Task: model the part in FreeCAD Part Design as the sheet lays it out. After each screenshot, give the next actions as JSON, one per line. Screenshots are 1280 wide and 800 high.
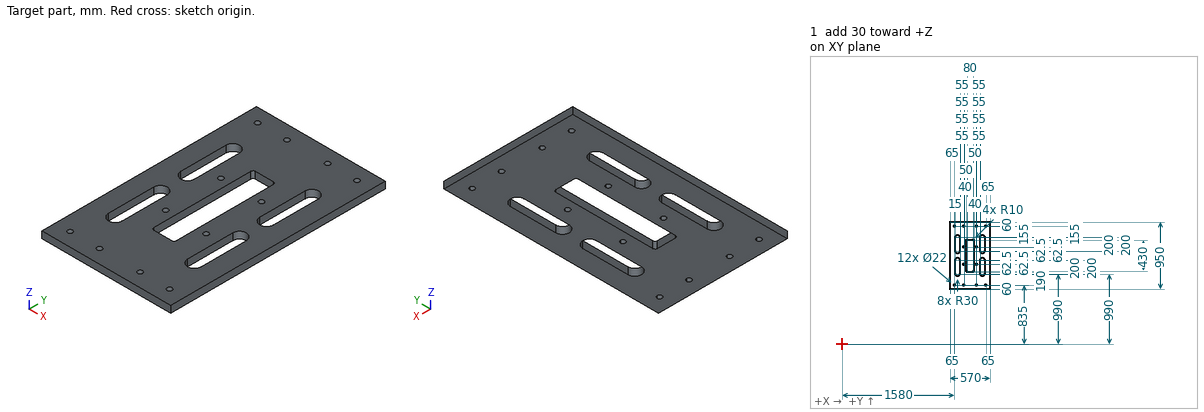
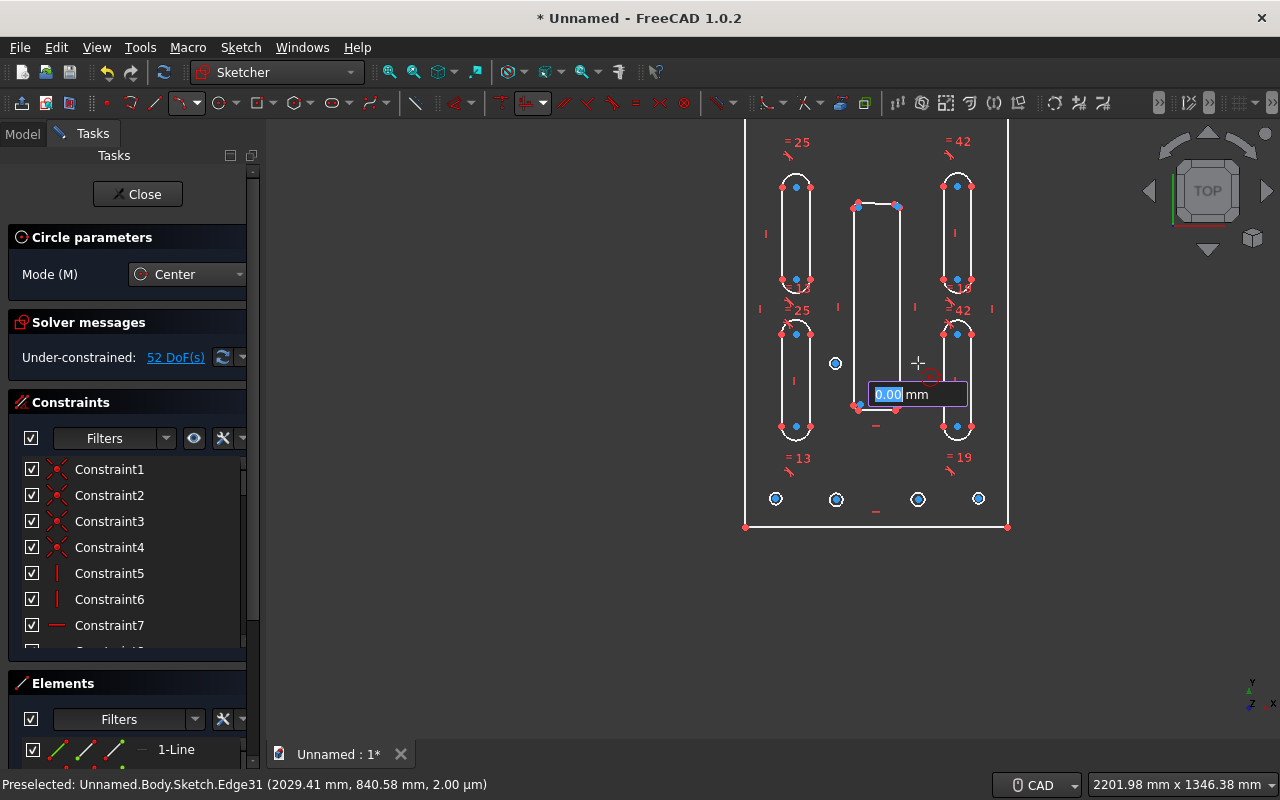
{"action": "scroll", "coordinate": [922, 359], "scroll_direction": "up", "scroll_amount": 6}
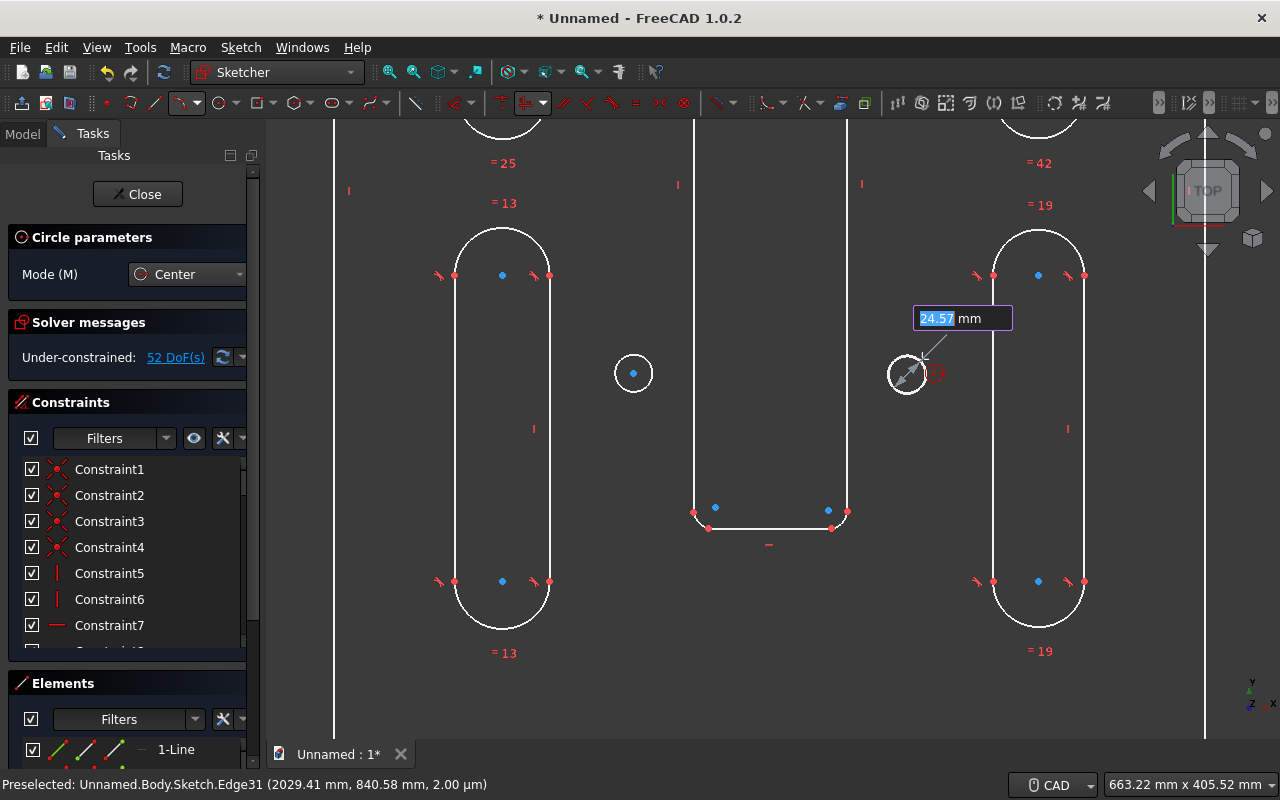
{"action": "left_click", "coordinate": [920, 358]}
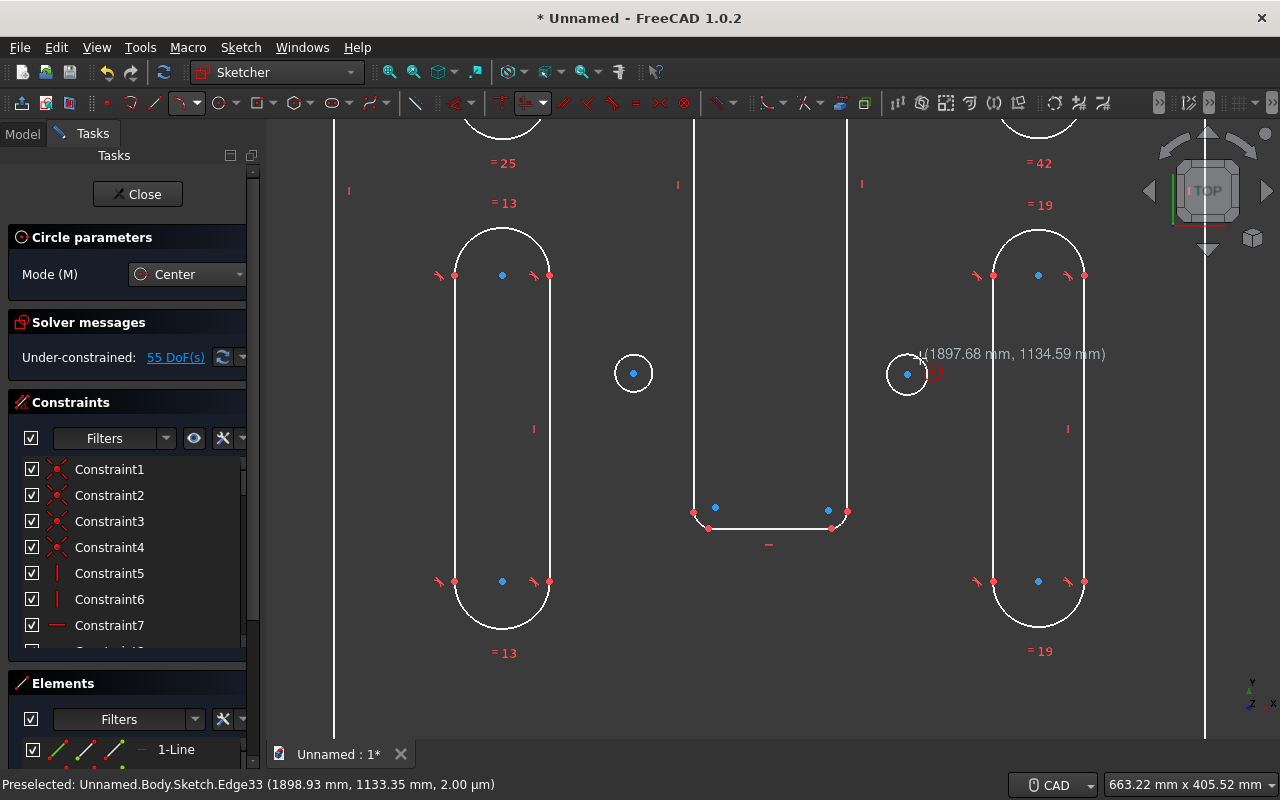
{"action": "scroll", "coordinate": [921, 360], "scroll_direction": "down", "scroll_amount": 9}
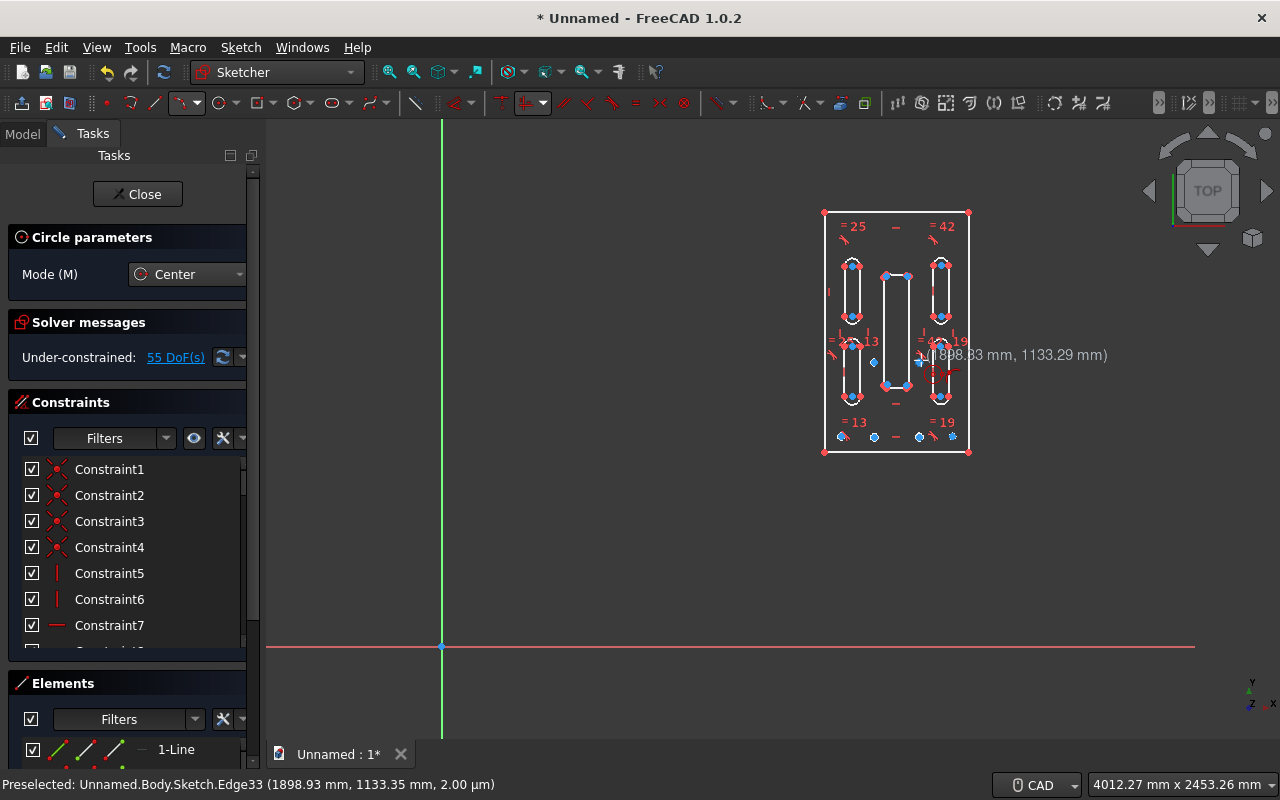
{"action": "scroll", "coordinate": [874, 300], "scroll_direction": "up", "scroll_amount": 11}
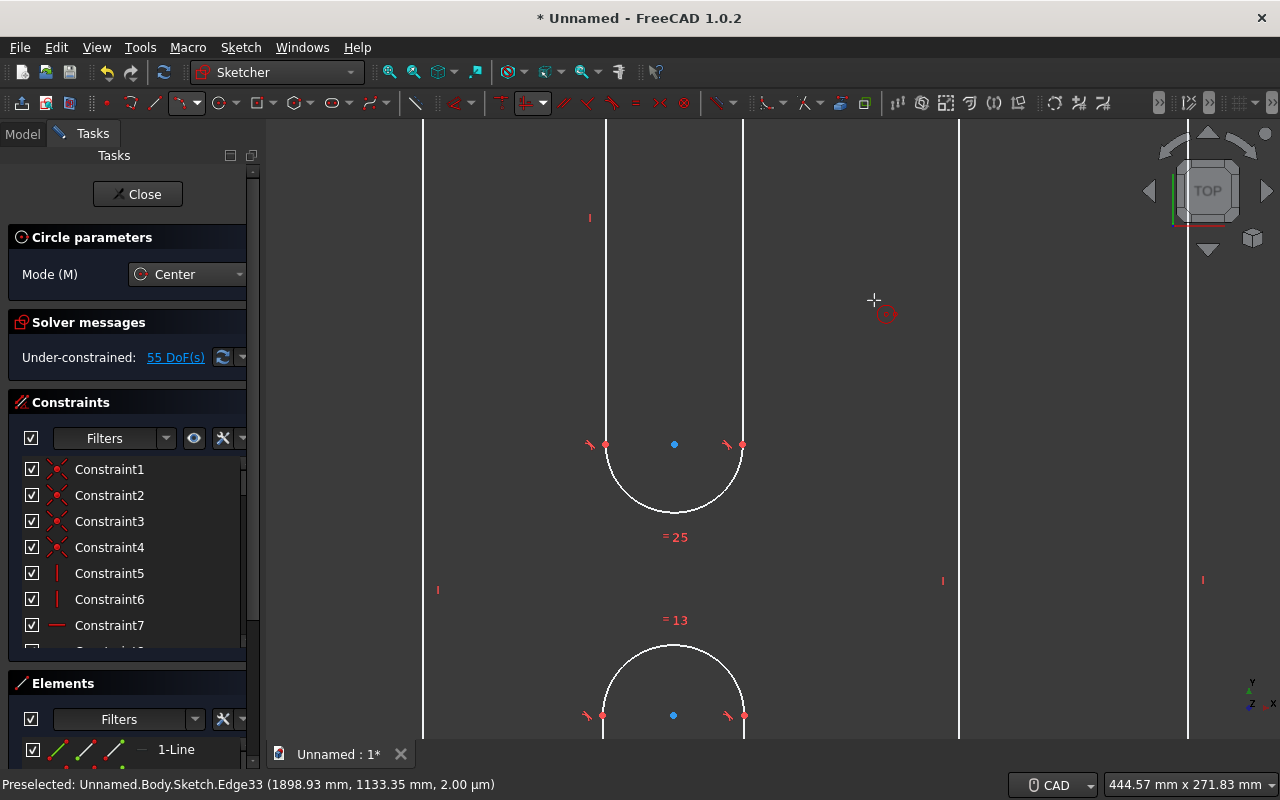
{"action": "scroll", "coordinate": [874, 300], "scroll_direction": "down", "scroll_amount": 11}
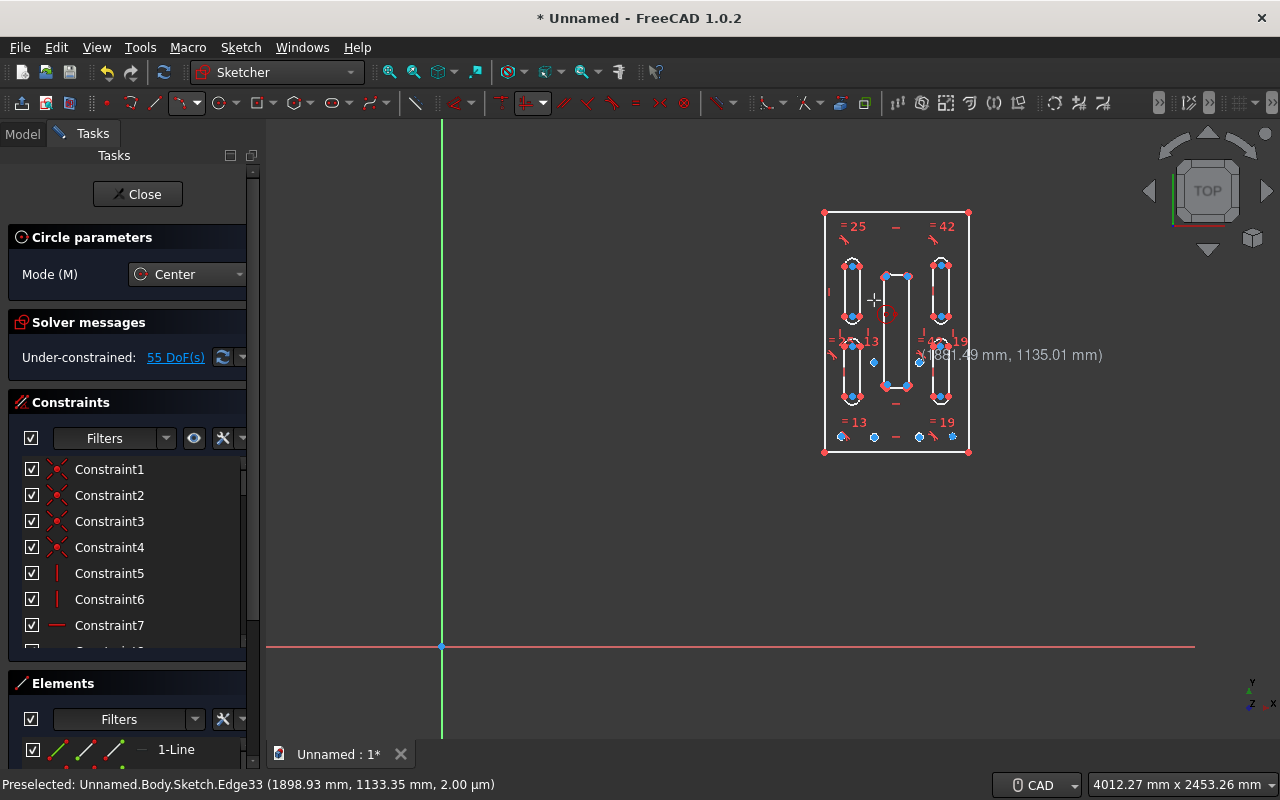
{"action": "scroll", "coordinate": [874, 300], "scroll_direction": "up", "scroll_amount": 3}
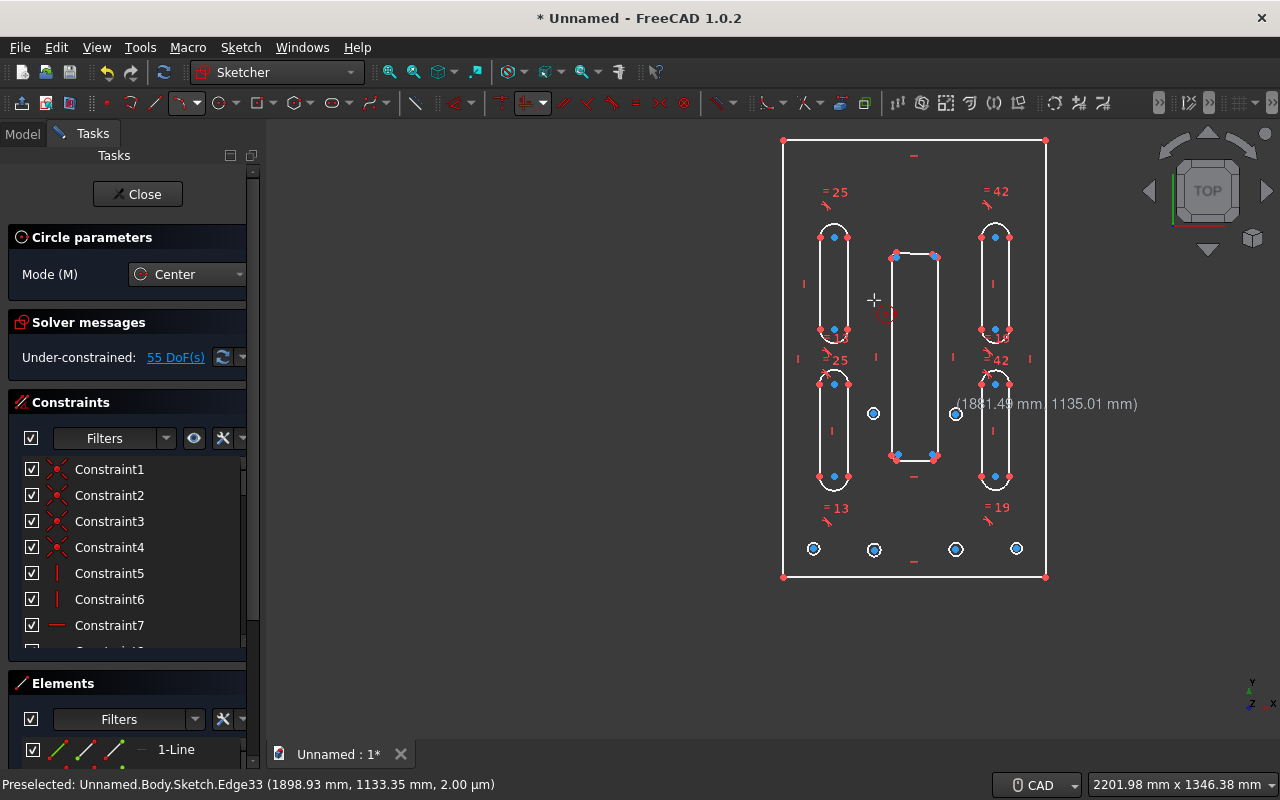
{"action": "left_click", "coordinate": [873, 300]}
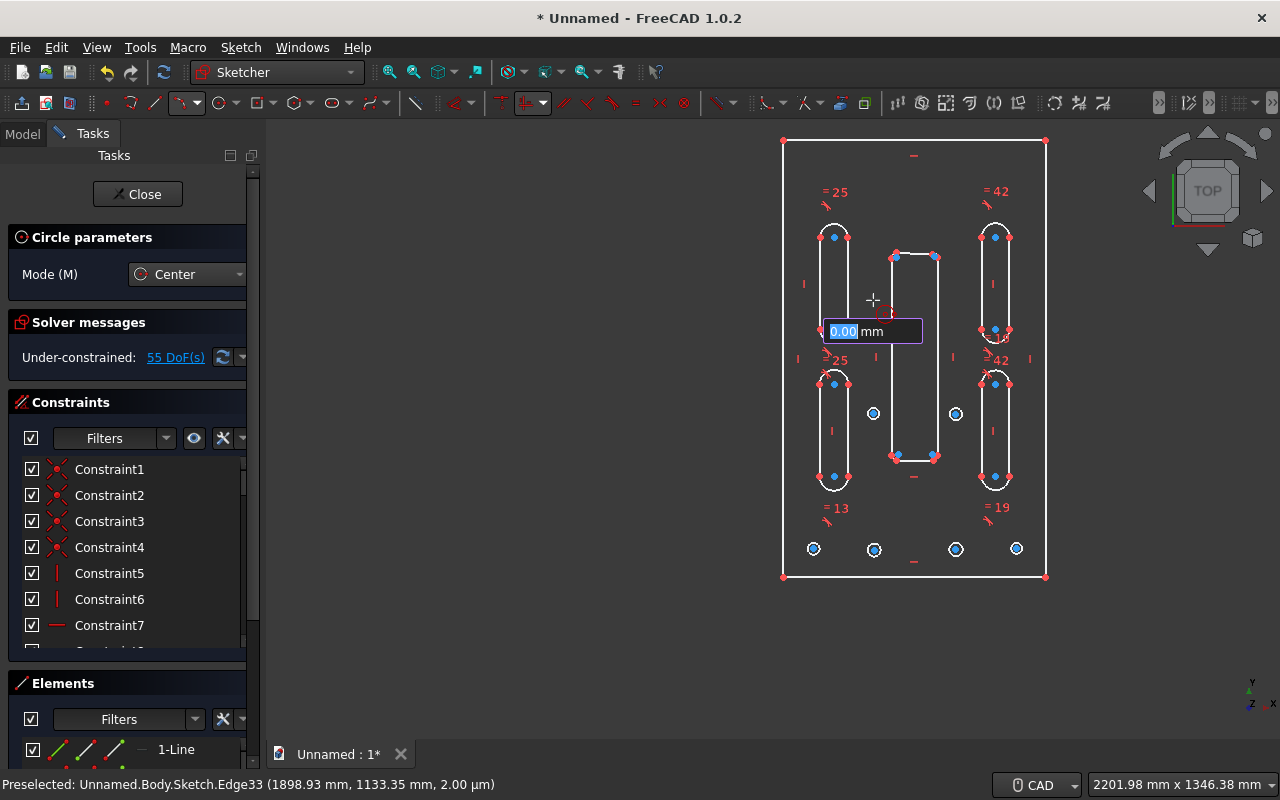
{"action": "scroll", "coordinate": [877, 296], "scroll_direction": "up", "scroll_amount": 6}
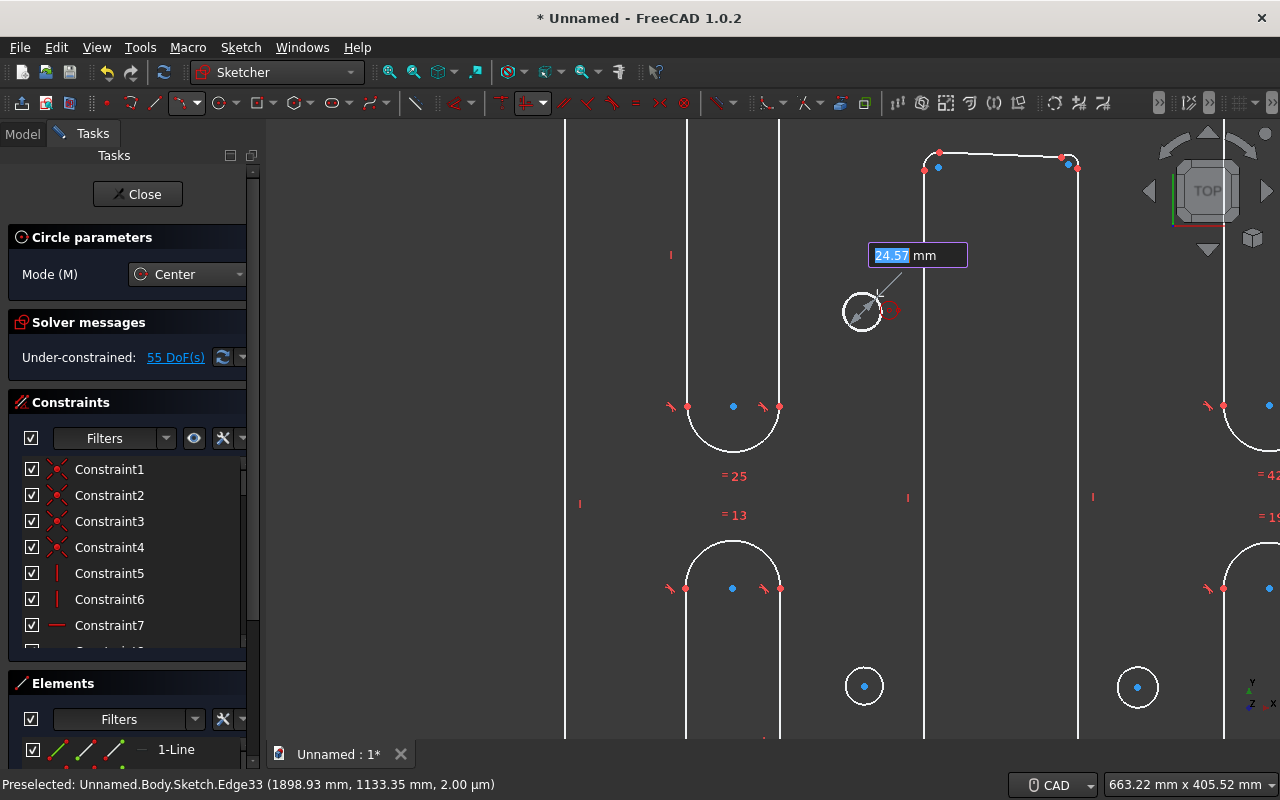
{"action": "left_click", "coordinate": [876, 296]}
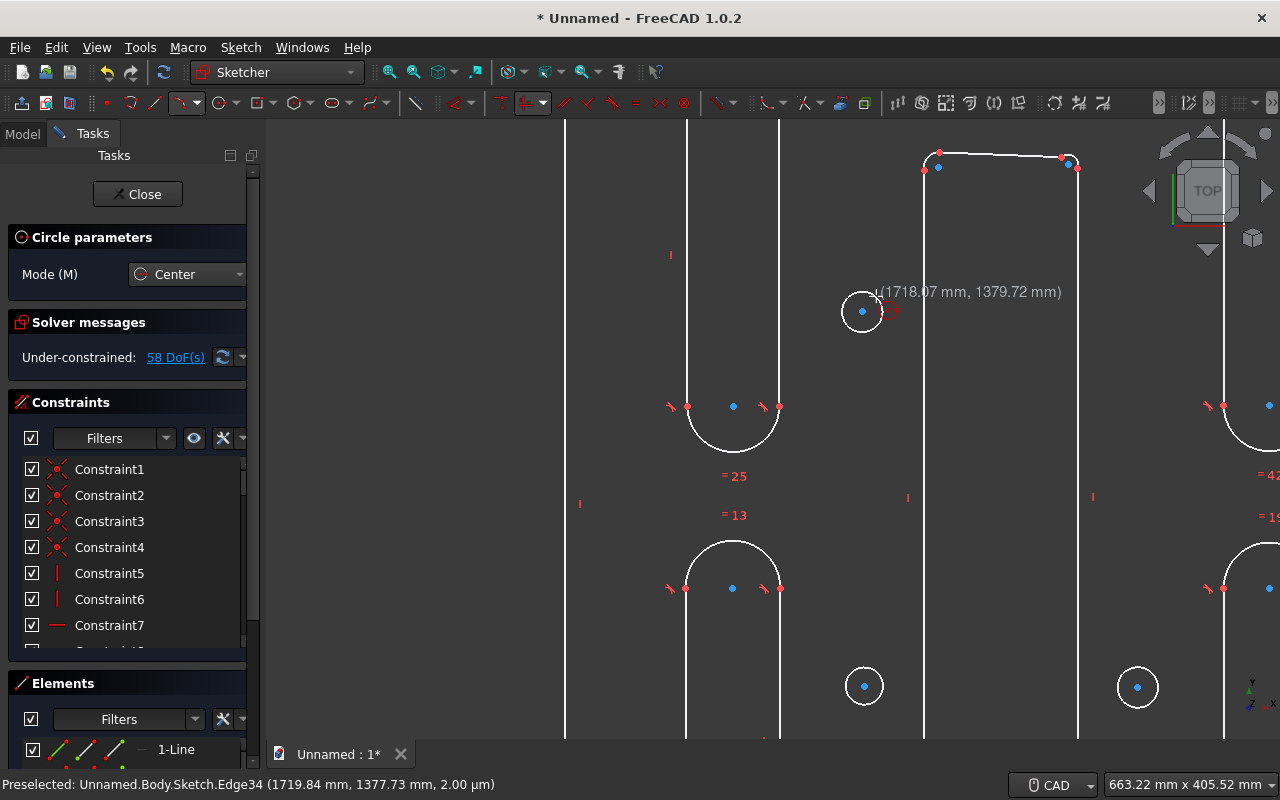
{"action": "scroll", "coordinate": [875, 299], "scroll_direction": "down", "scroll_amount": 9}